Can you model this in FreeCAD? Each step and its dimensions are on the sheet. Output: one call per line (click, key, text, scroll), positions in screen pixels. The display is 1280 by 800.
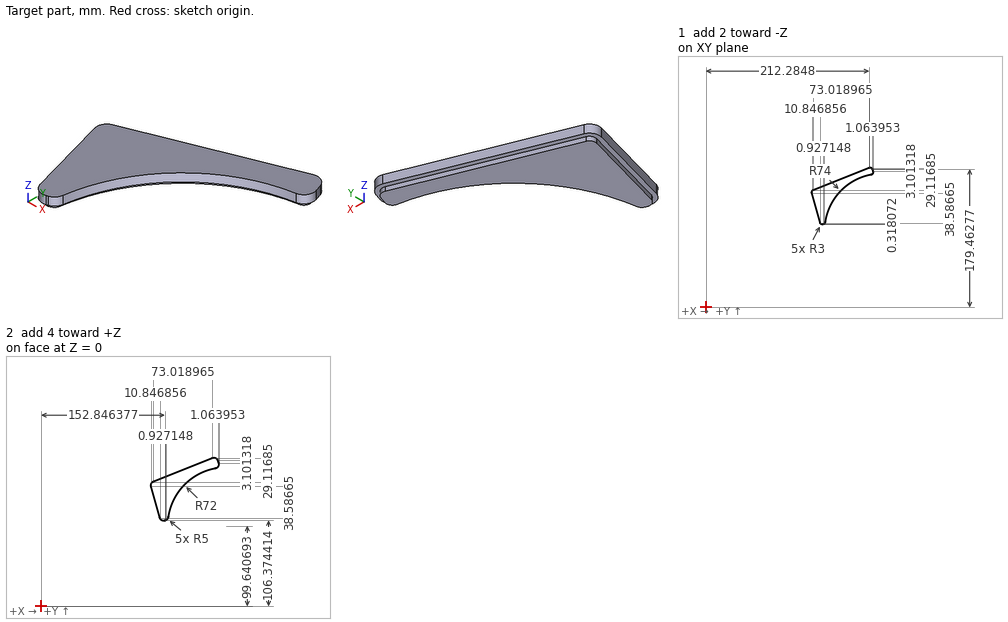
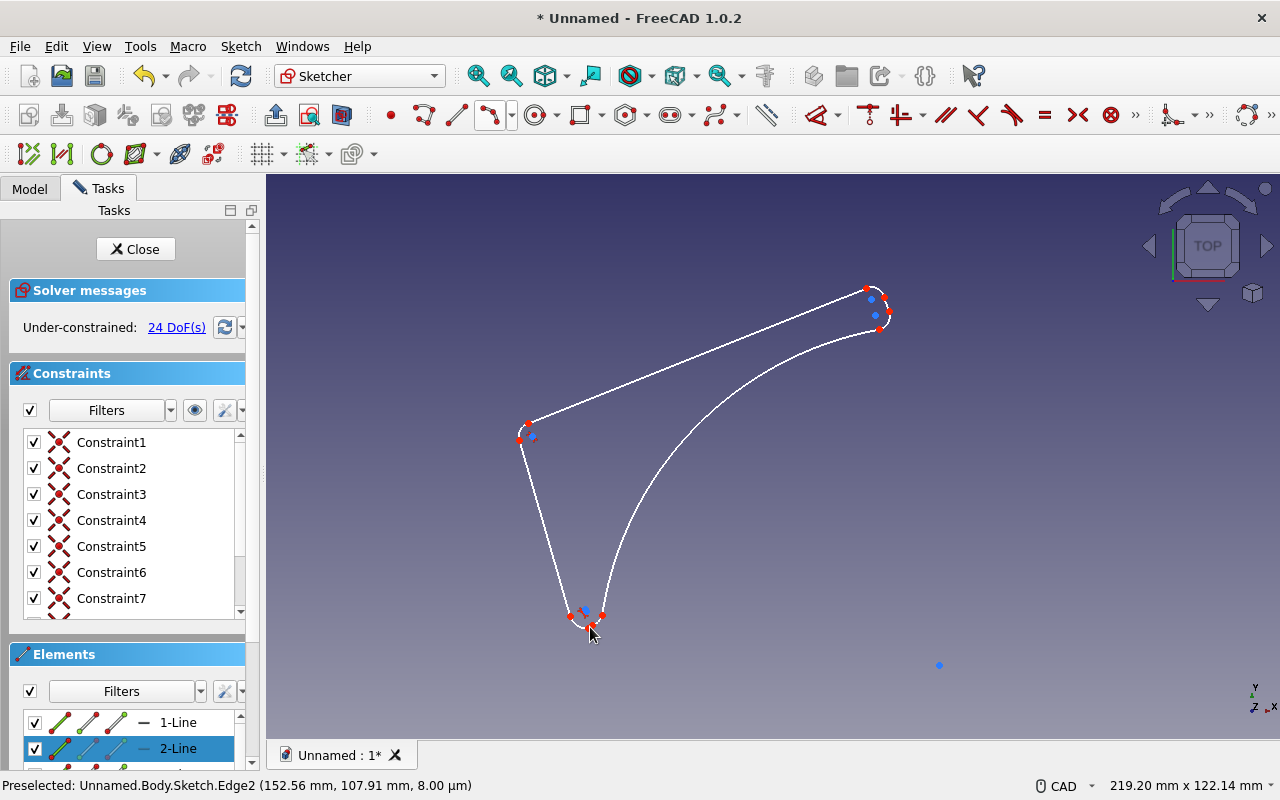
scroll(573, 622, up, 4)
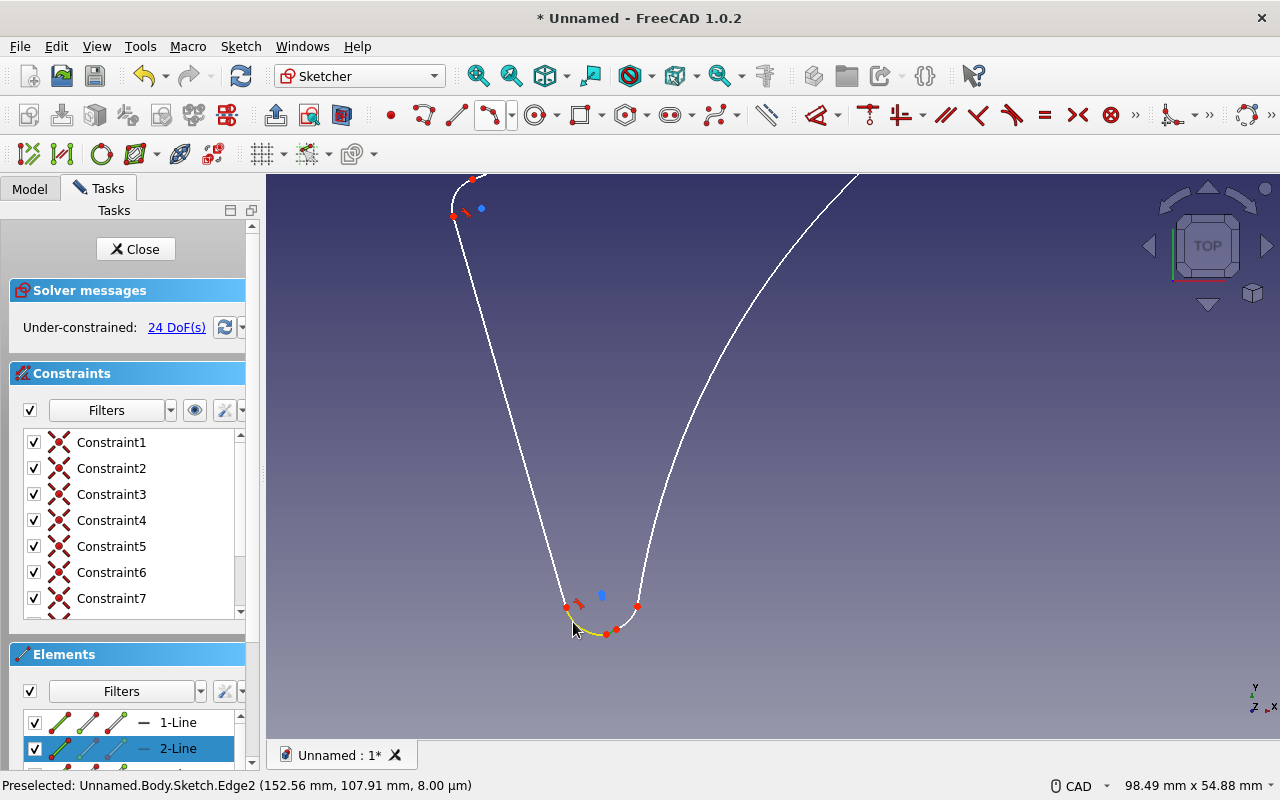
click(574, 622)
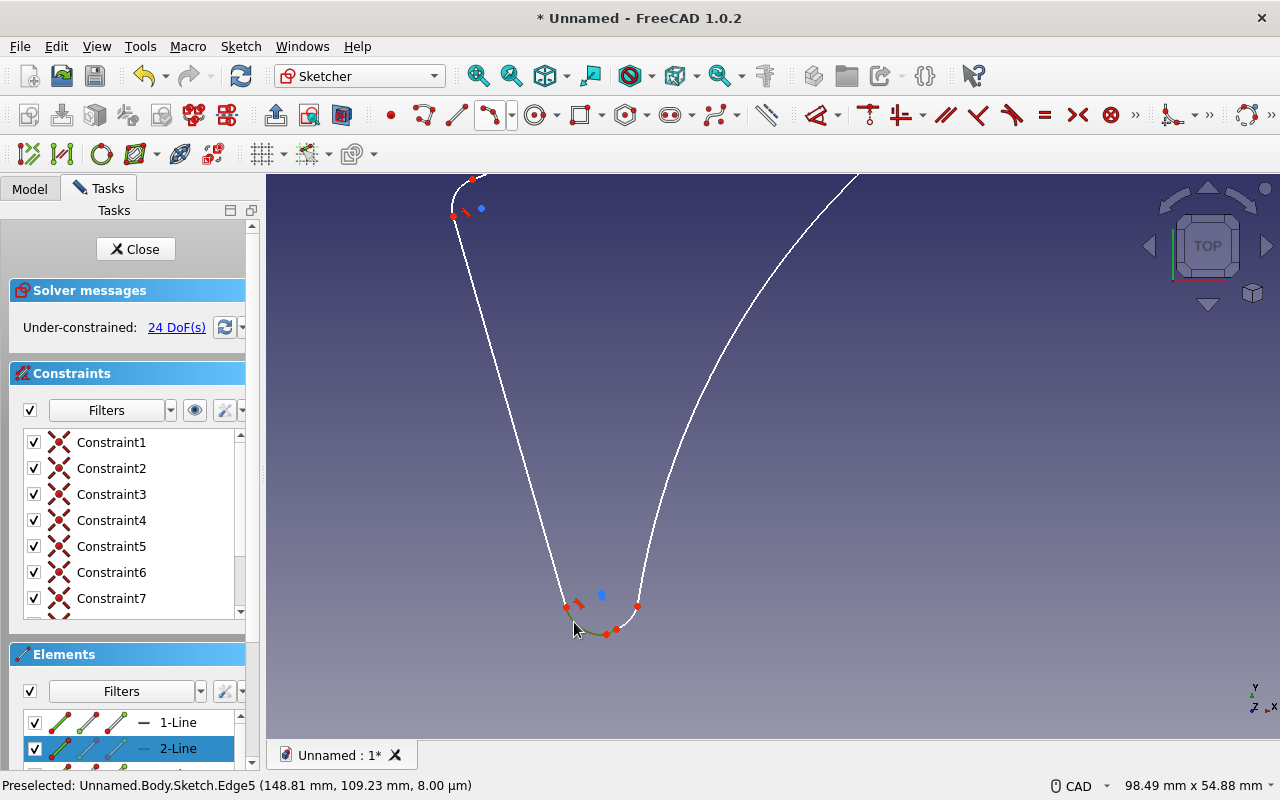
click(1012, 116)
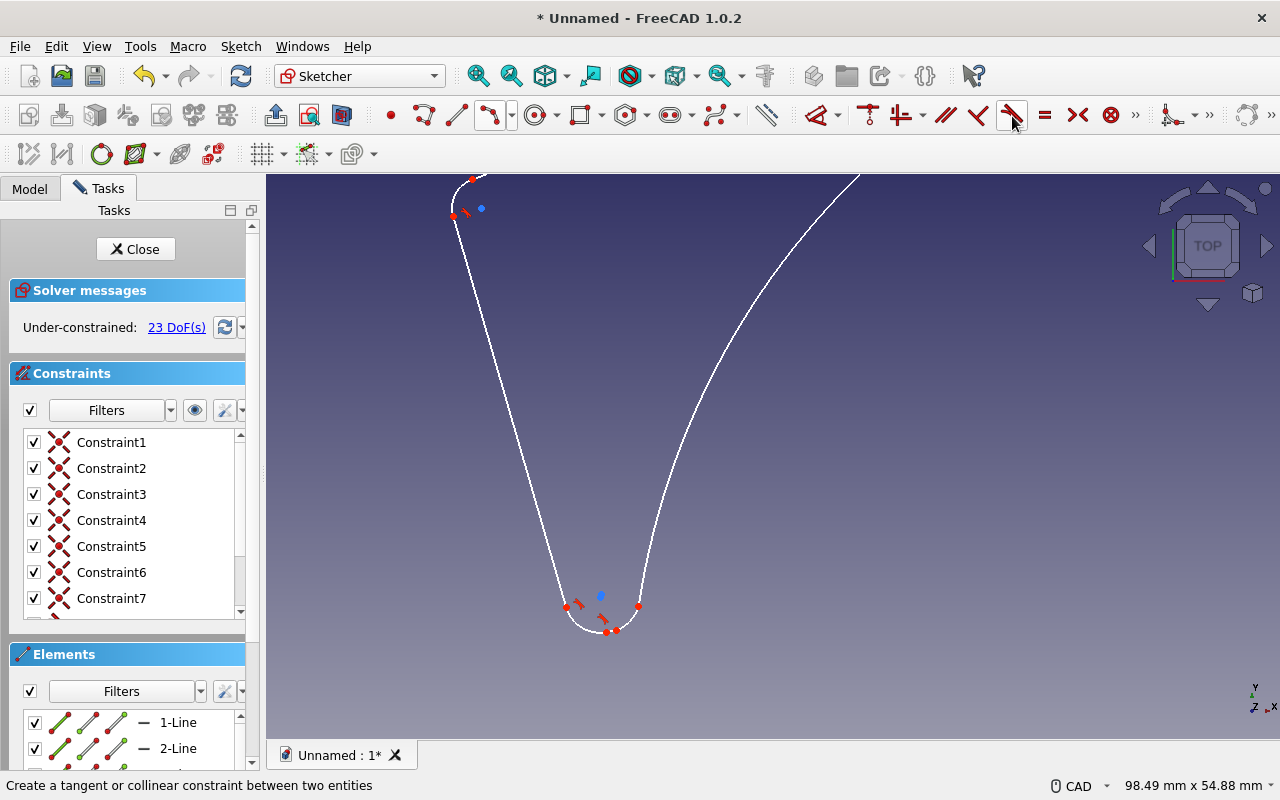
scroll(611, 631, up, 5)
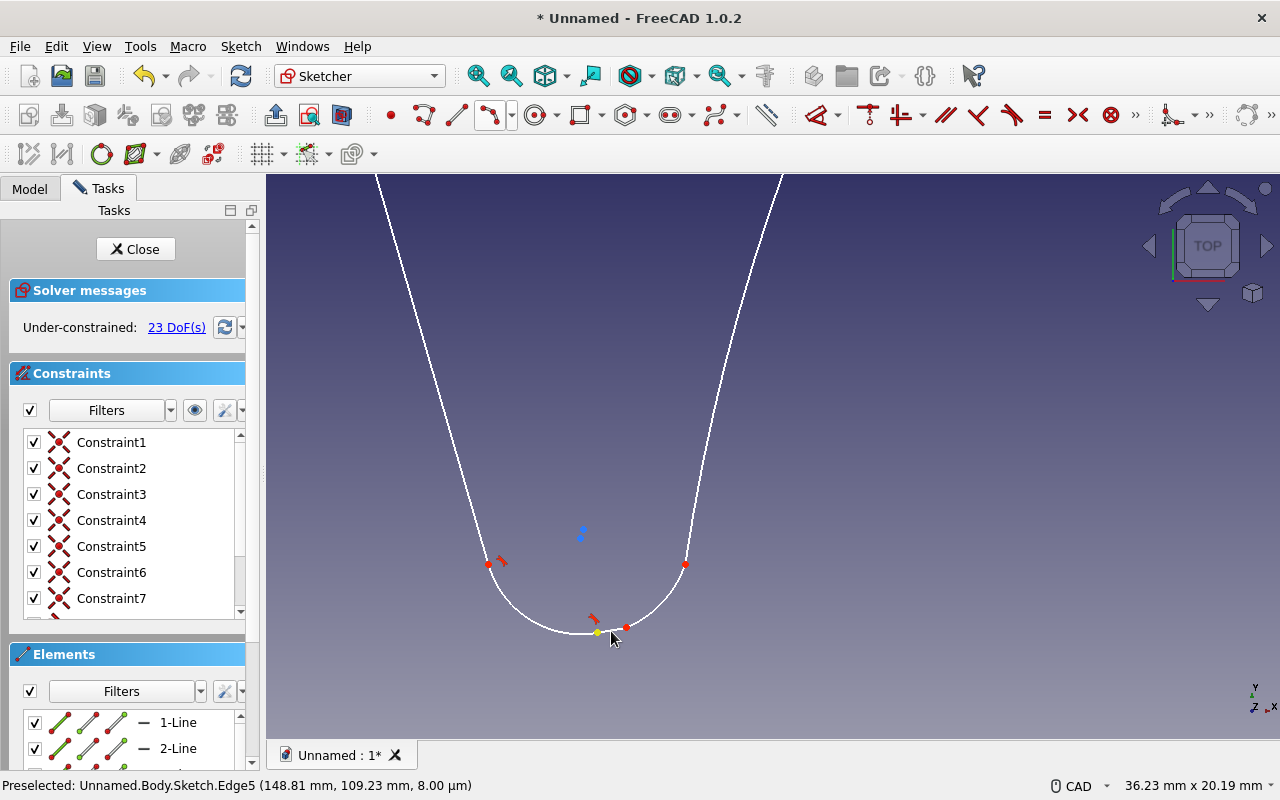
click(612, 630)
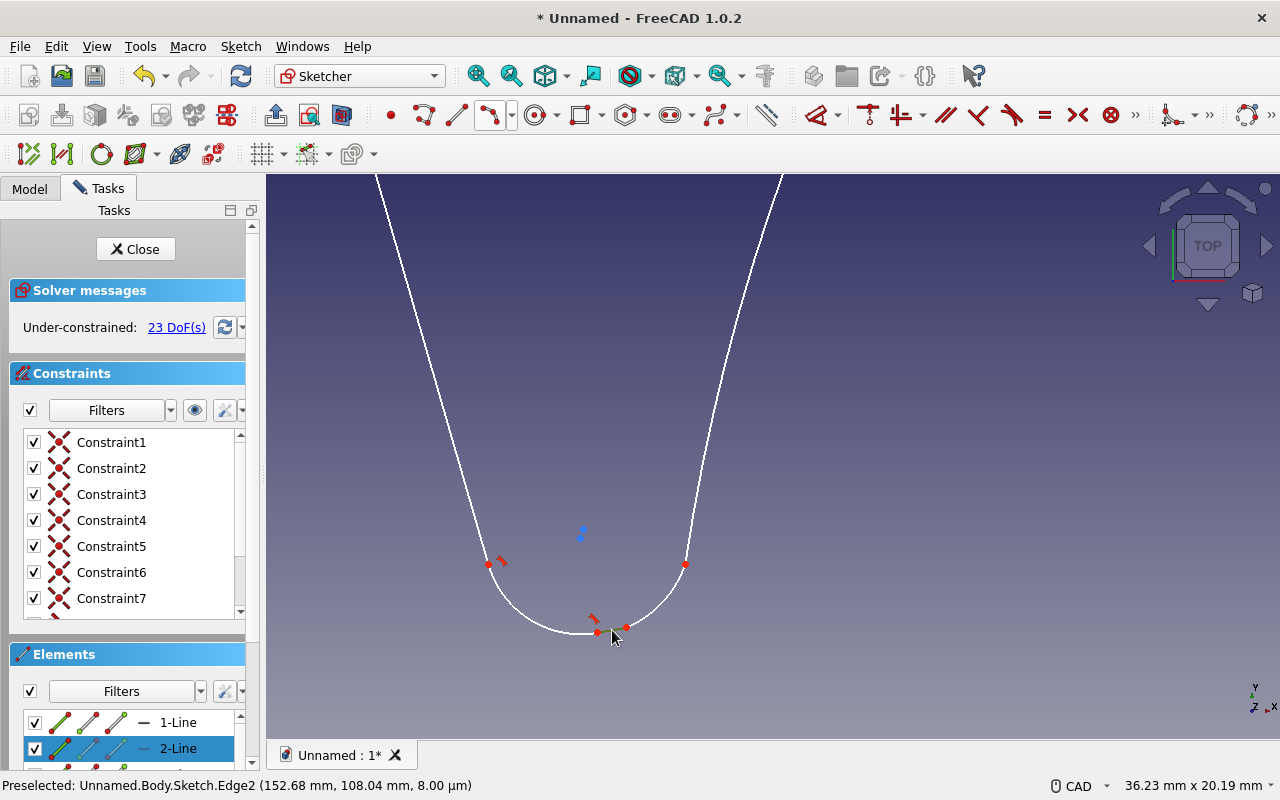
click(649, 614)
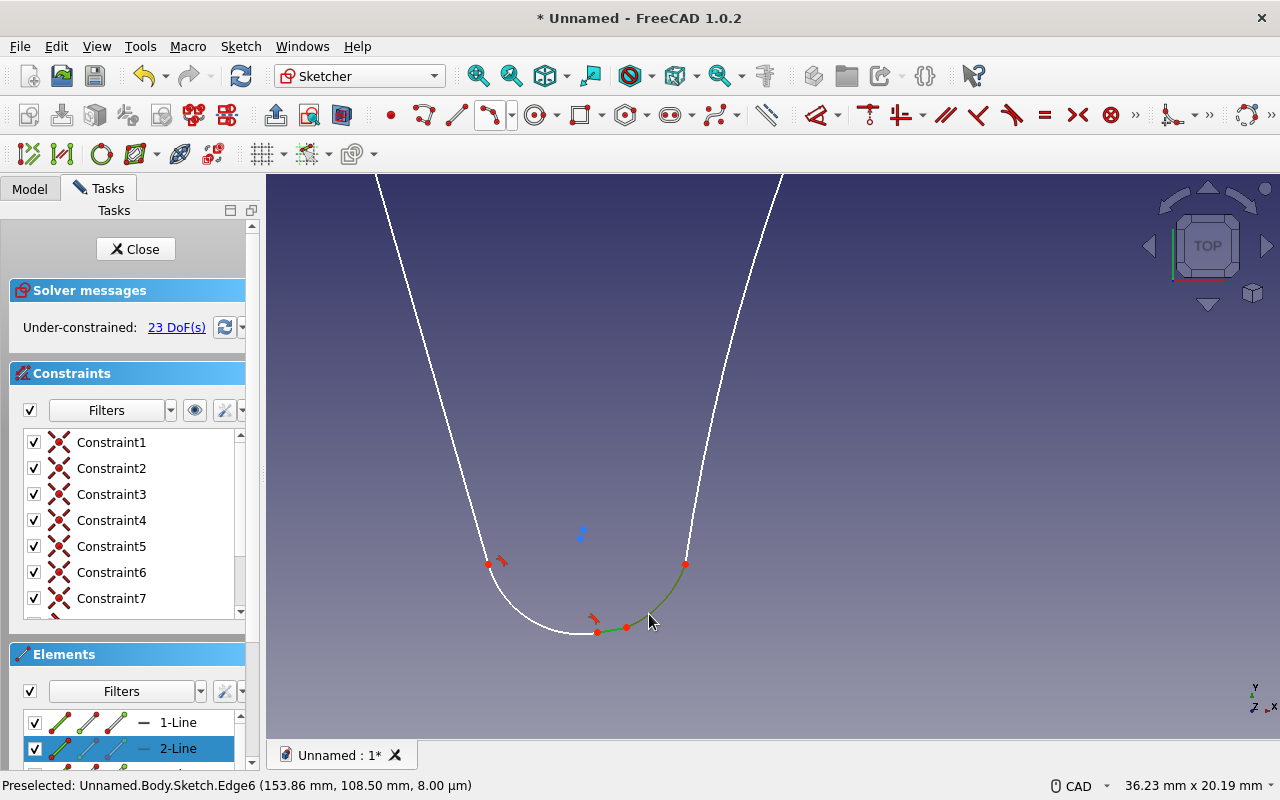
click(1012, 116)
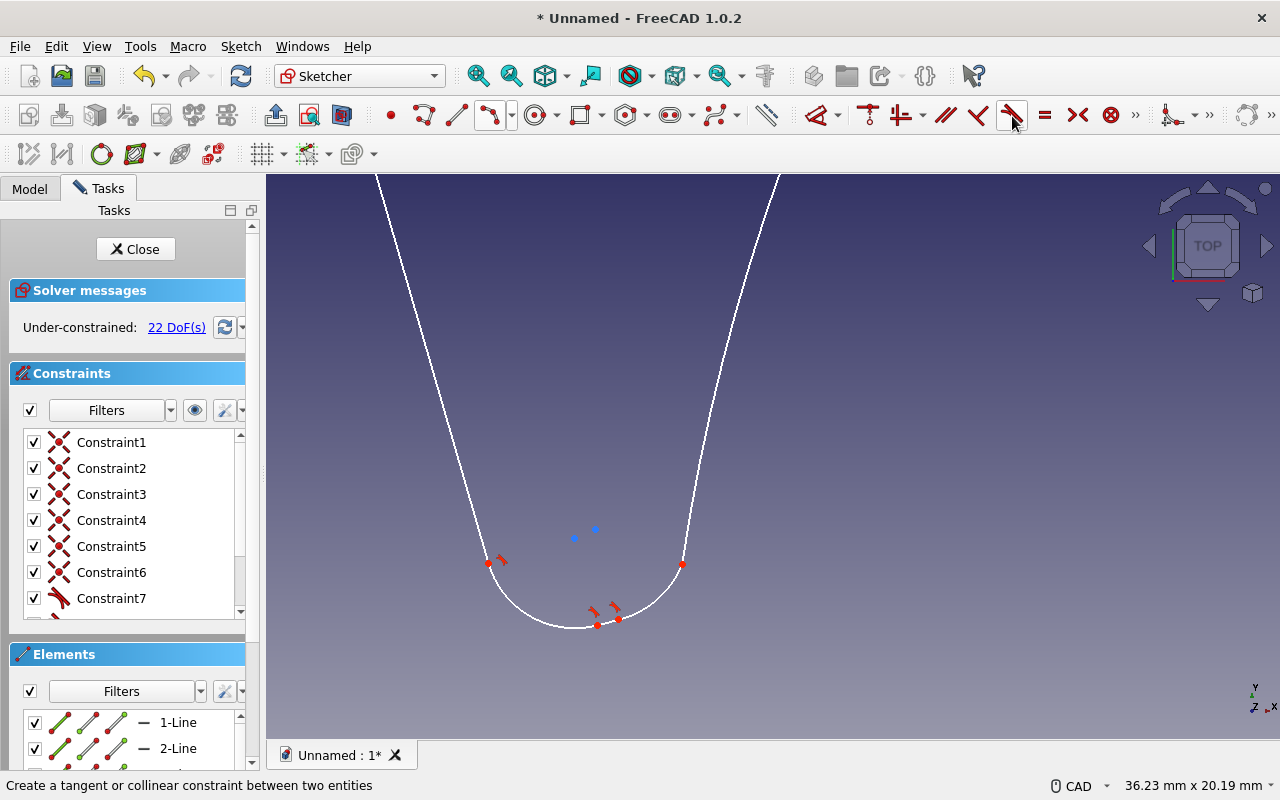
scroll(586, 625, down, 9)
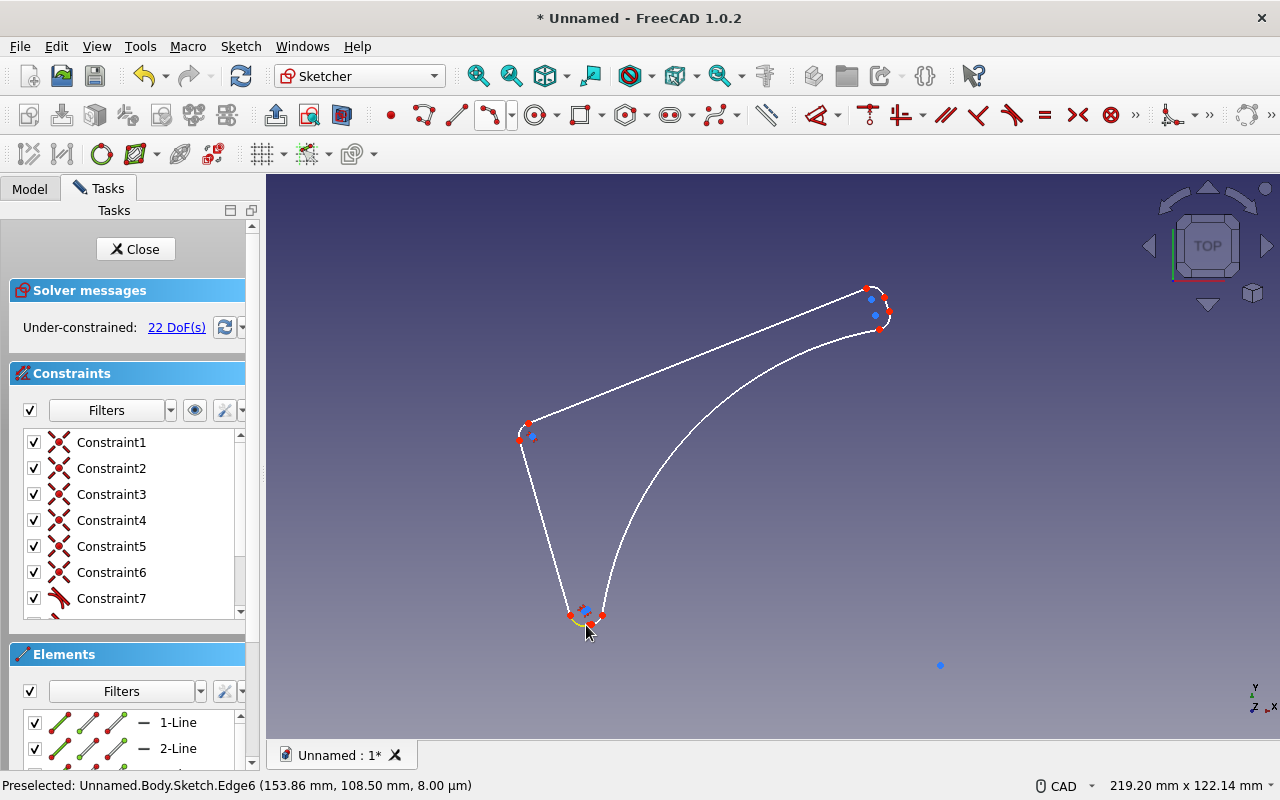
scroll(888, 307, up, 6)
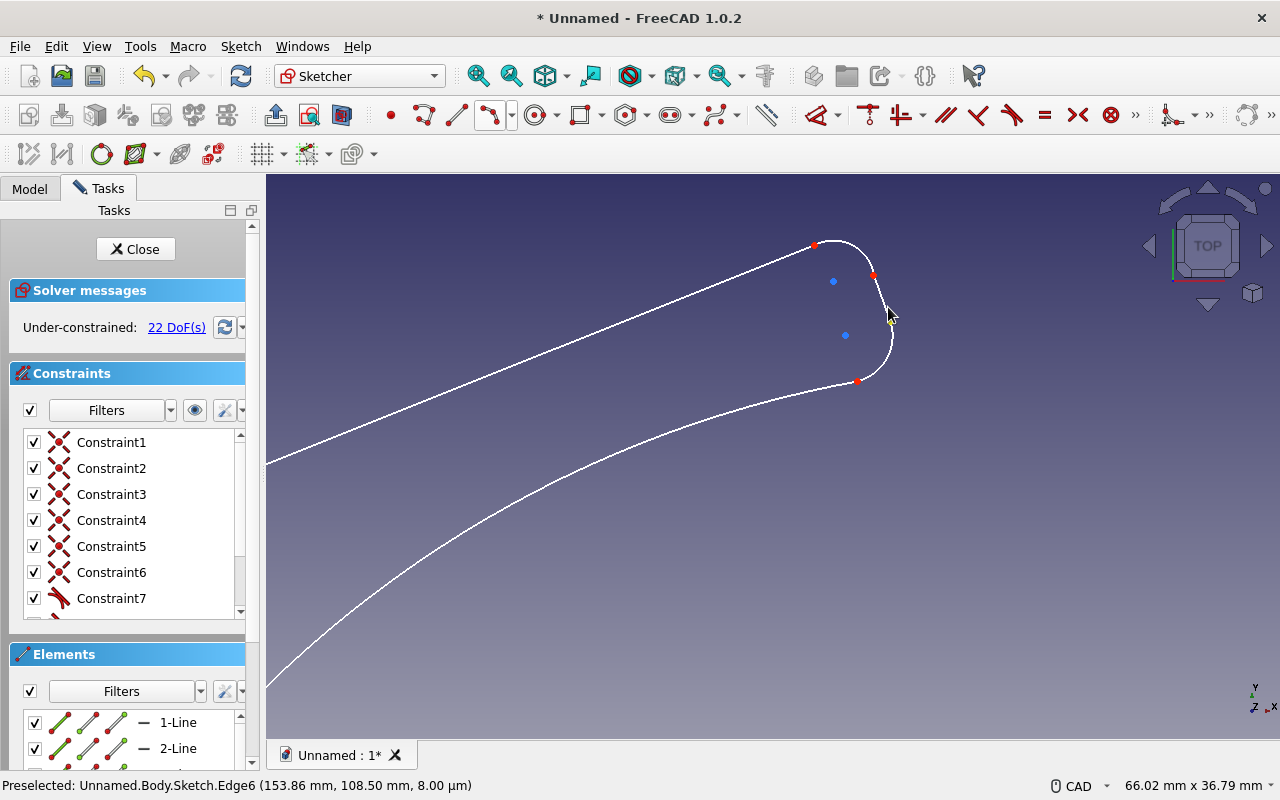
click(886, 308)